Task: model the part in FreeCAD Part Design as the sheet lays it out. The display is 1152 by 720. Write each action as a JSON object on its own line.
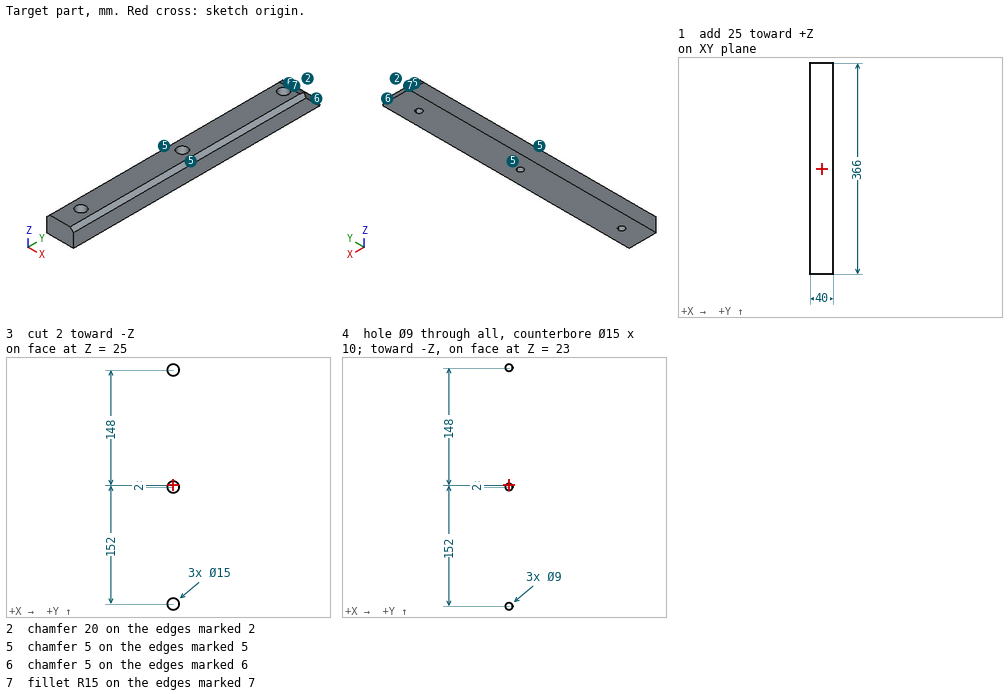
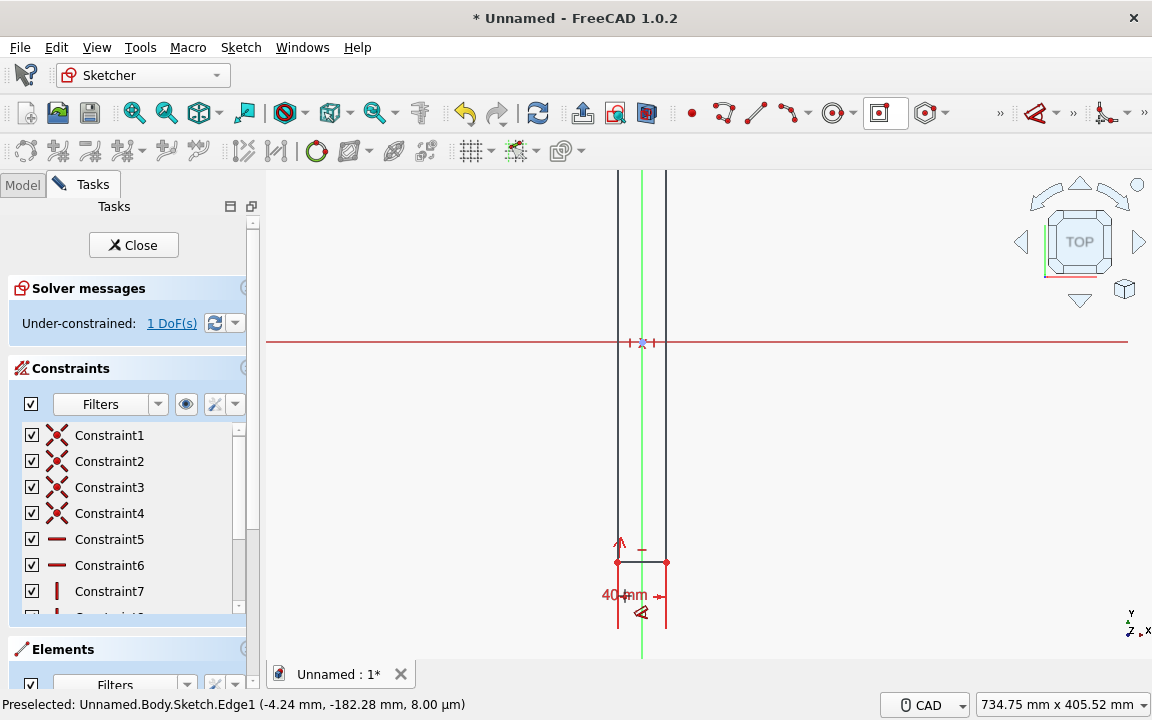
{"action": "left_click", "coordinate": [666, 430]}
{"action": "left_click", "coordinate": [700, 380]}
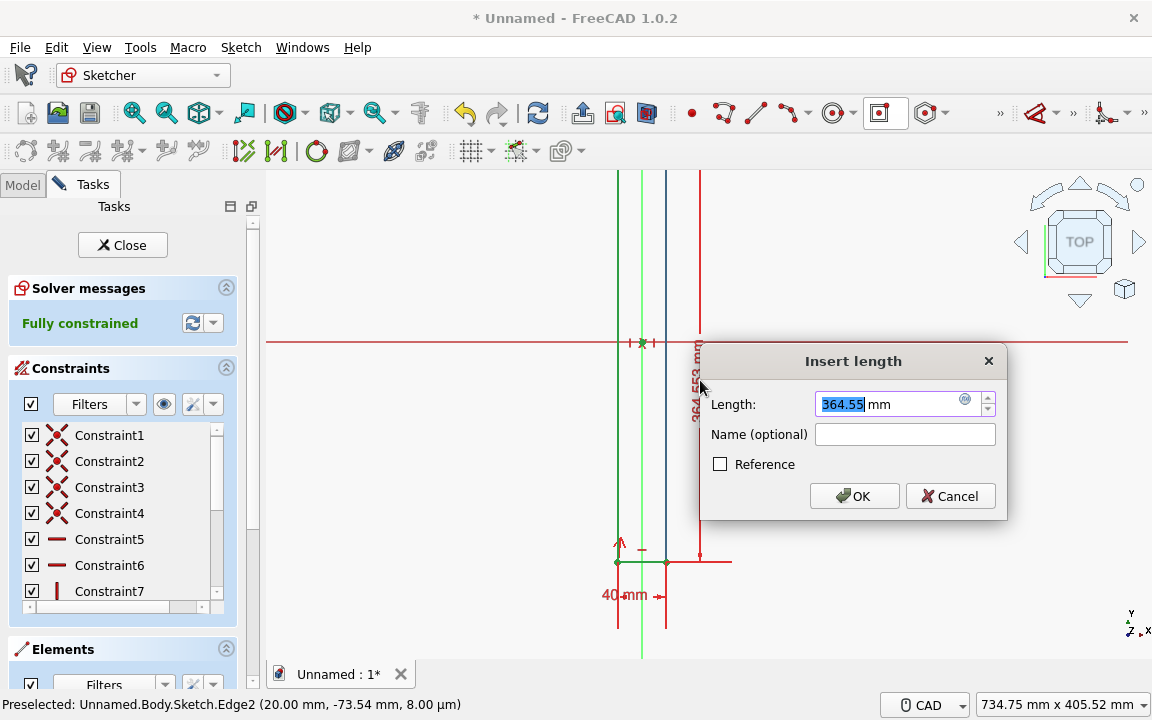
{"action": "type", "text": "366"}
{"action": "key", "text": "Return"}
{"action": "key", "text": "Escape"}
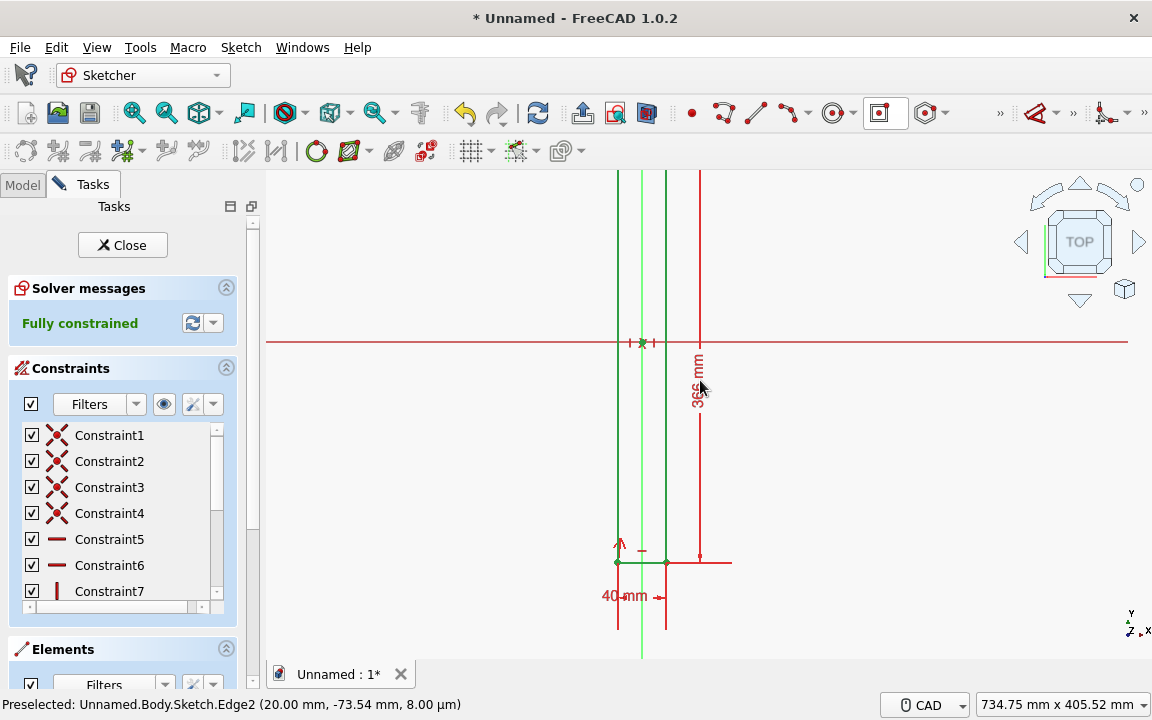
{"action": "left_click", "coordinate": [123, 245]}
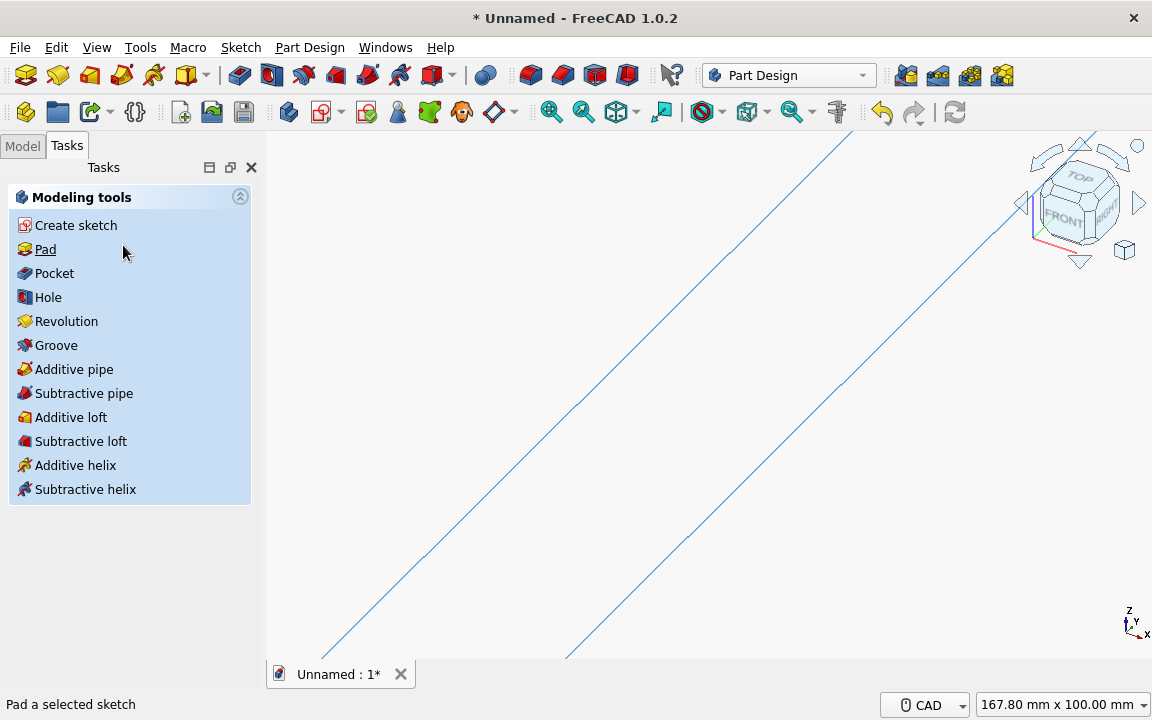
{"action": "left_click", "coordinate": [26, 76]}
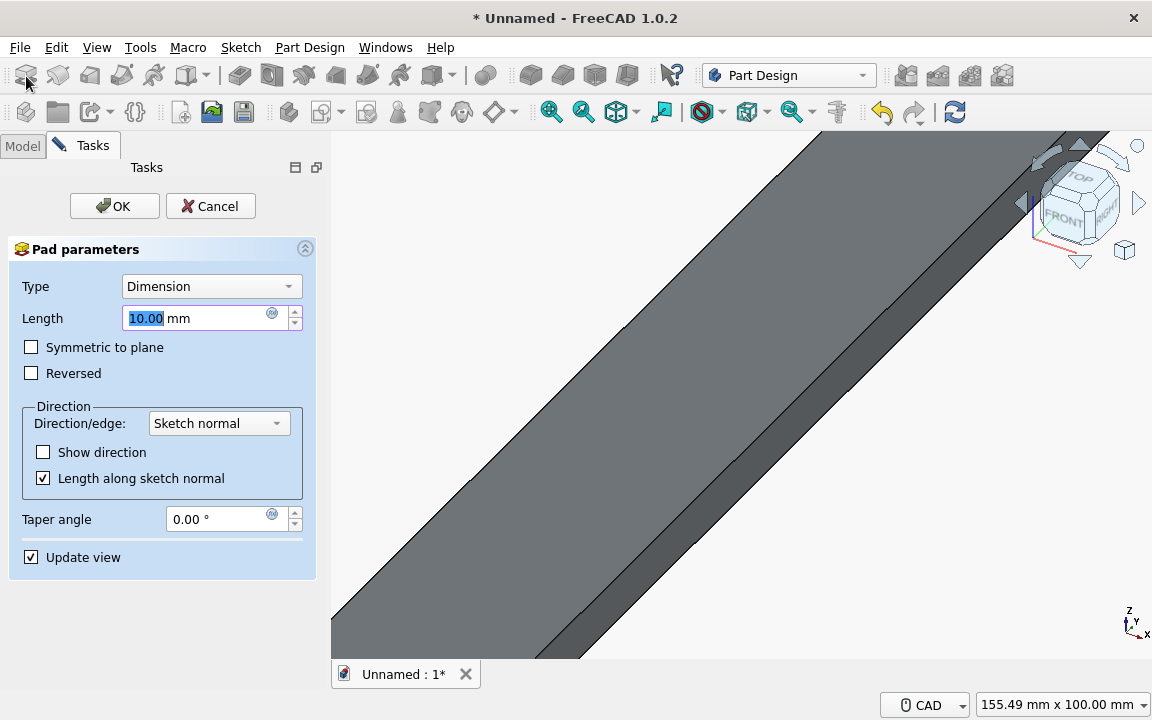
{"action": "type", "text": "25"}
{"action": "key", "text": "Tab"}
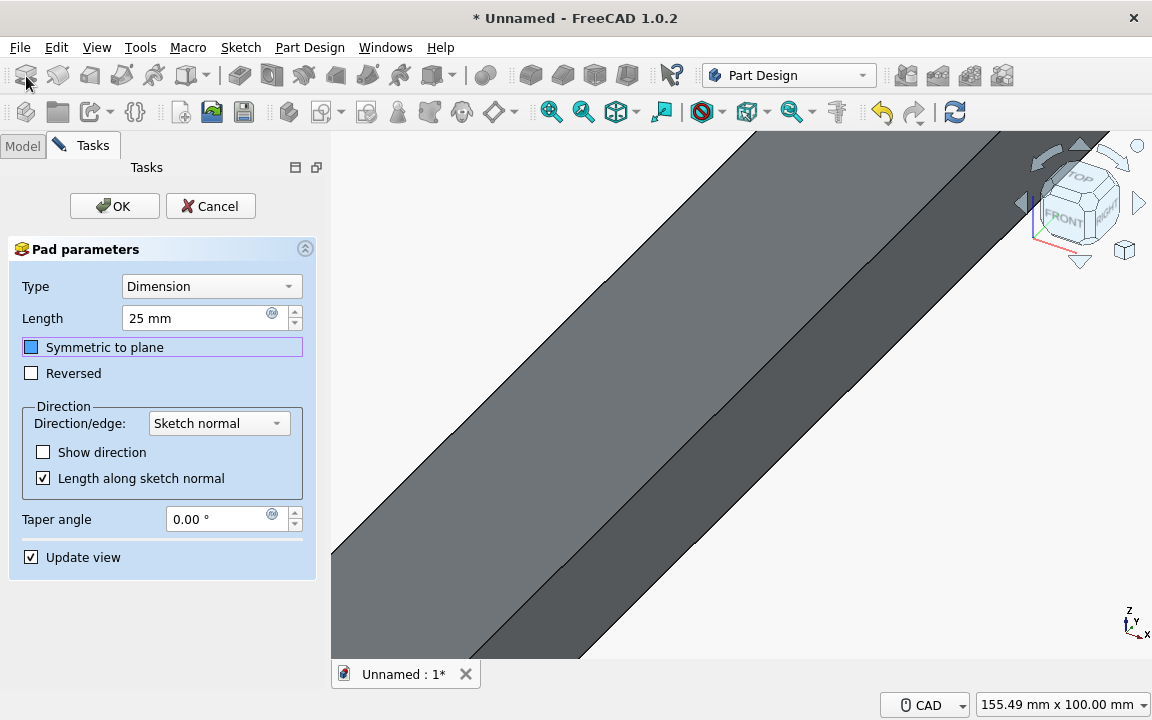
{"action": "left_click", "coordinate": [115, 206]}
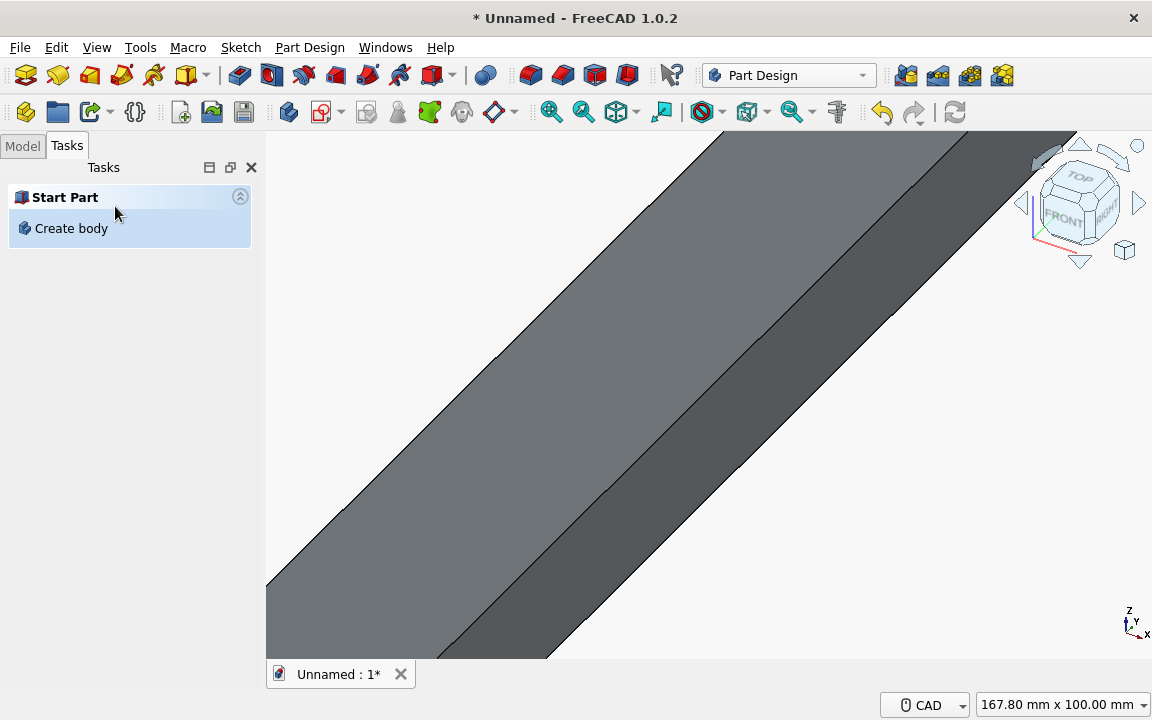
{"action": "key", "text": "v f"}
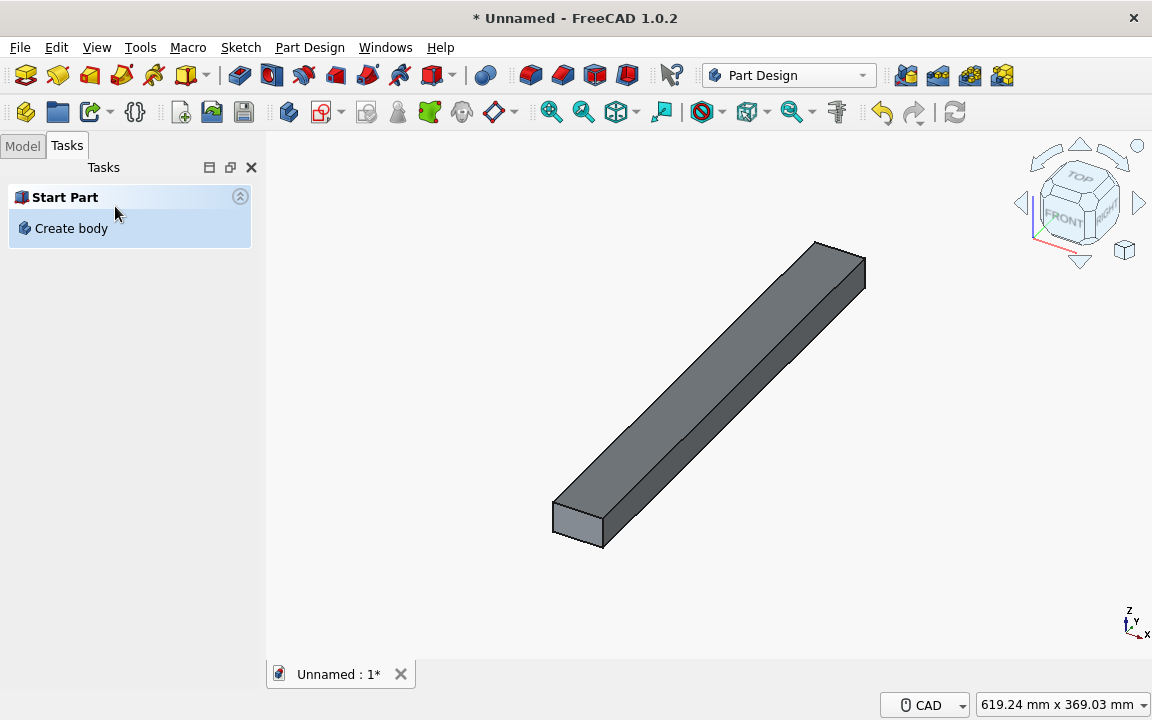
{"action": "key", "text": "0"}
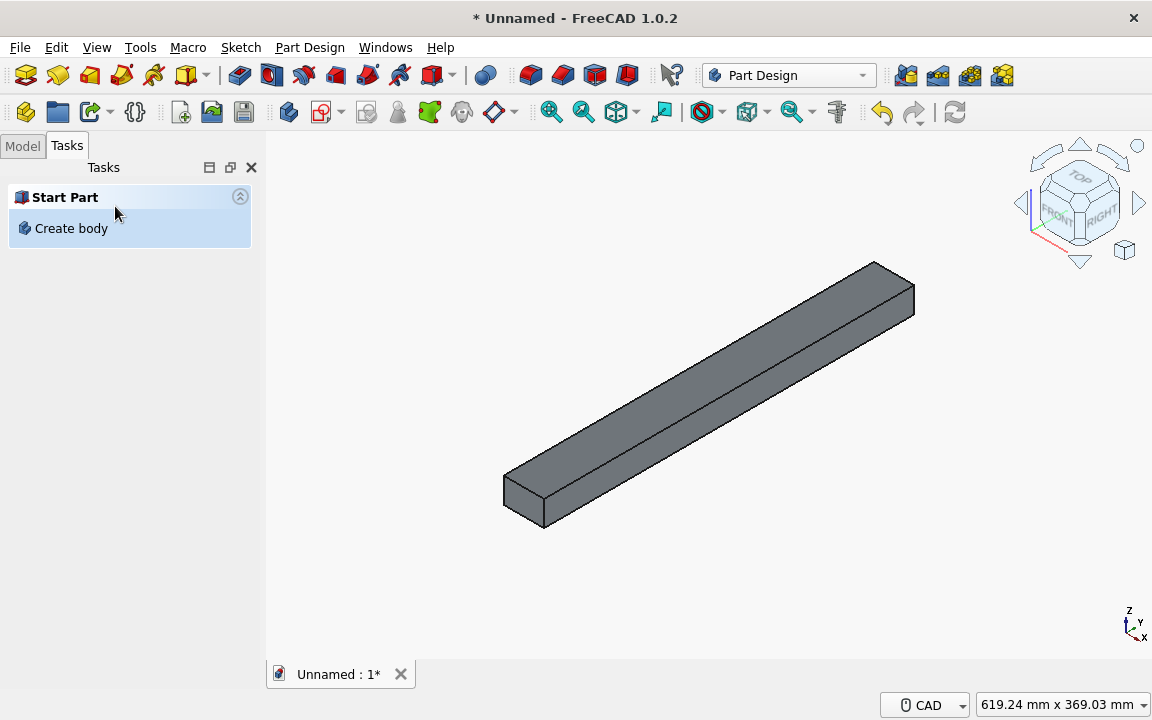
{"action": "key", "text": "2"}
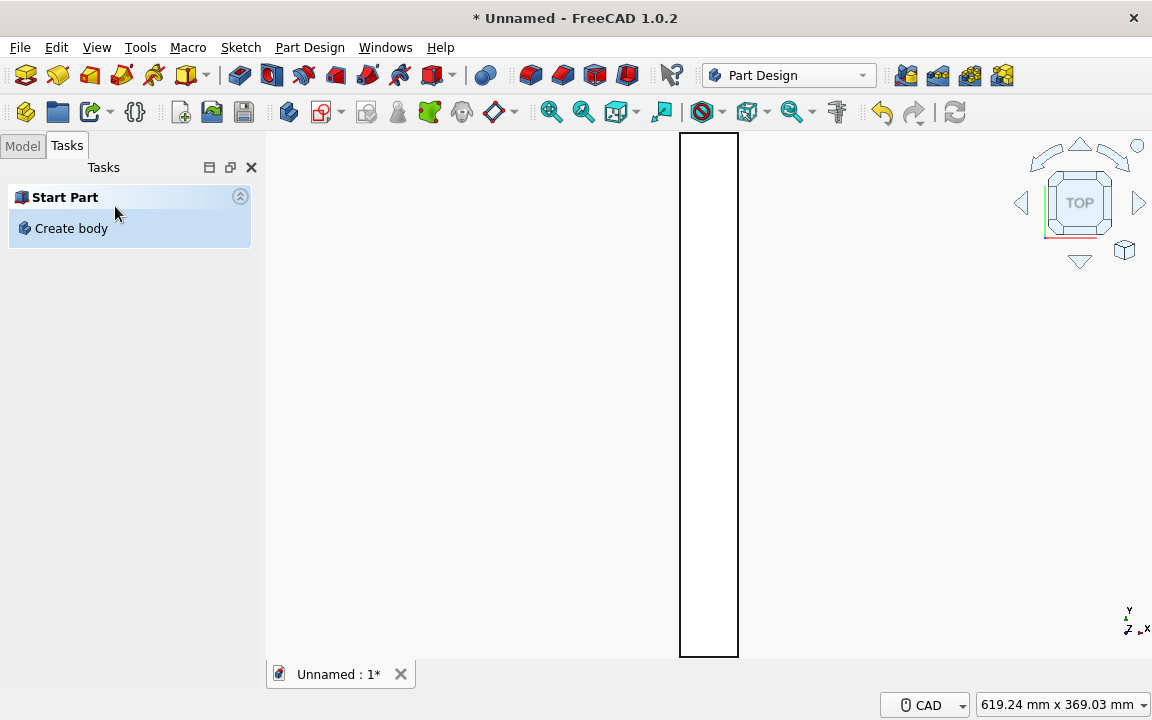
{"action": "key", "text": "1"}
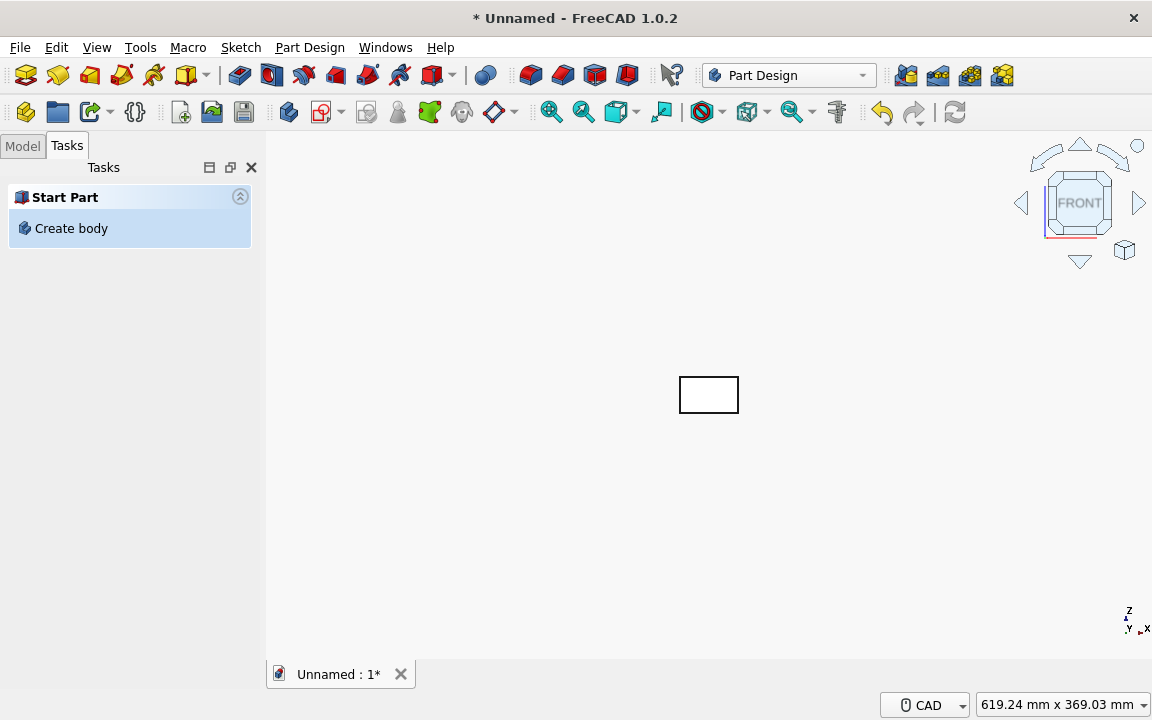
{"action": "left_click", "coordinate": [552, 112]}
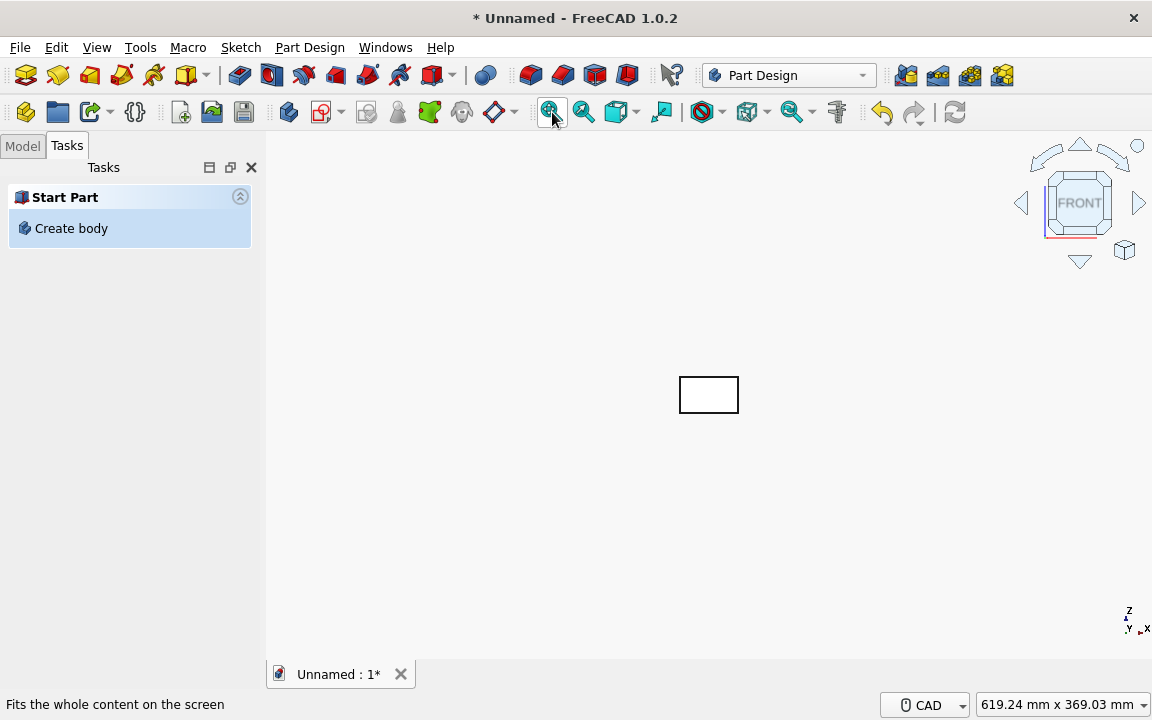
{"action": "key", "text": "3"}